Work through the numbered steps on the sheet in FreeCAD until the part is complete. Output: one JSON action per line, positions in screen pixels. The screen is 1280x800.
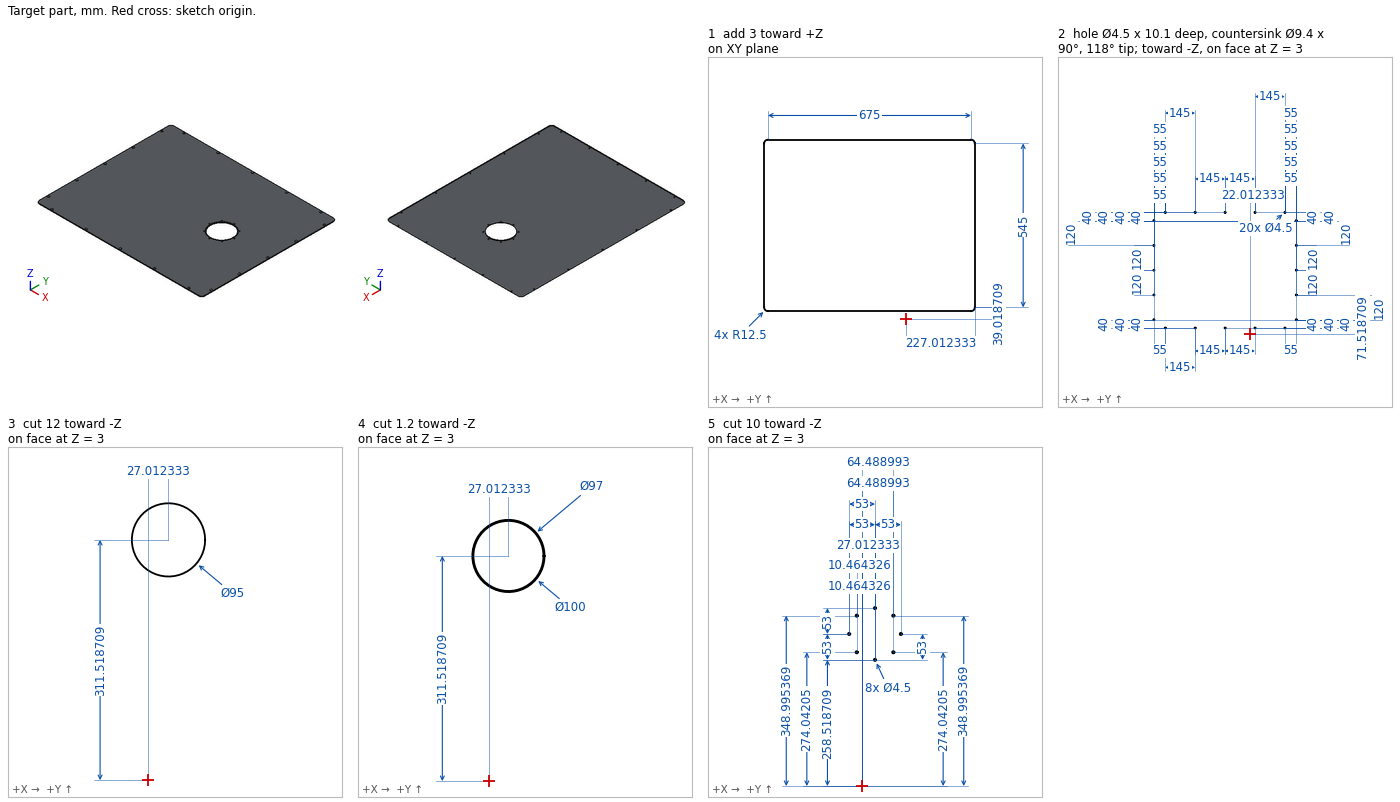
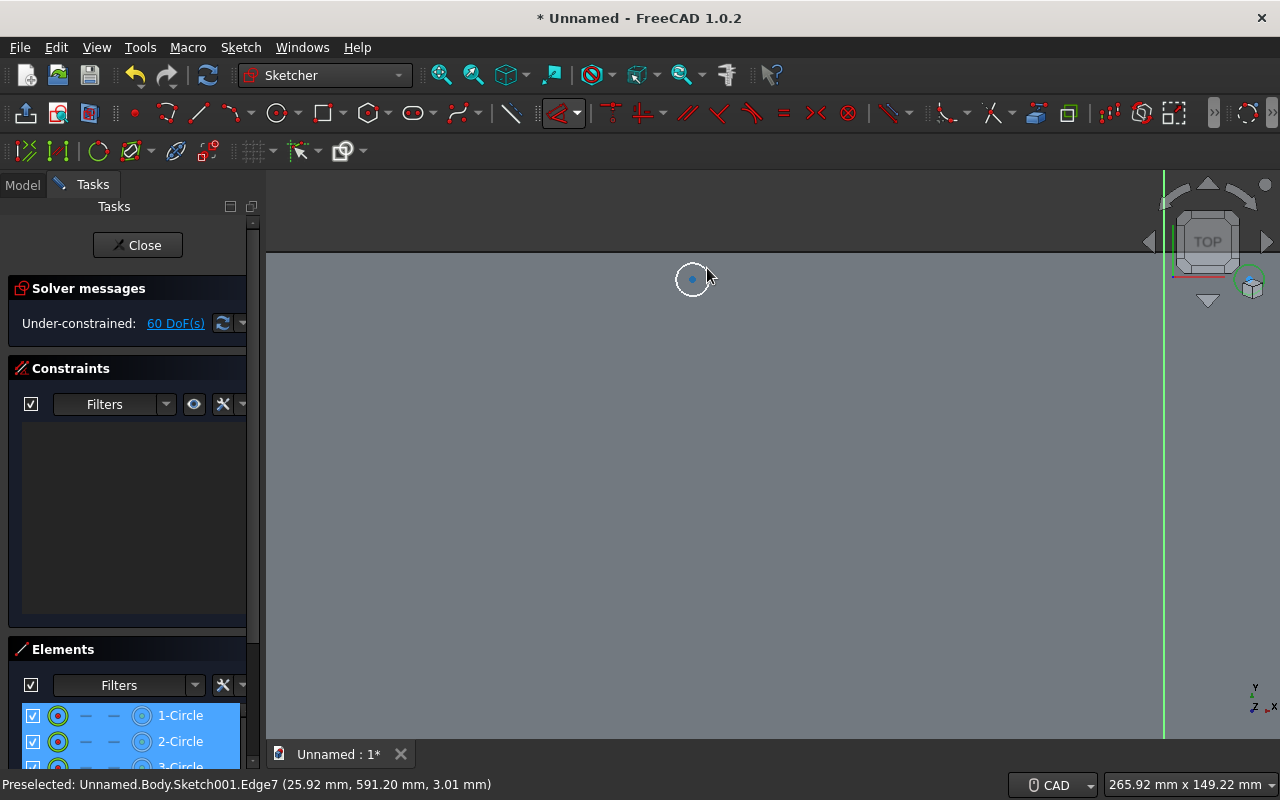
{"action": "left_click", "coordinate": [704, 268]}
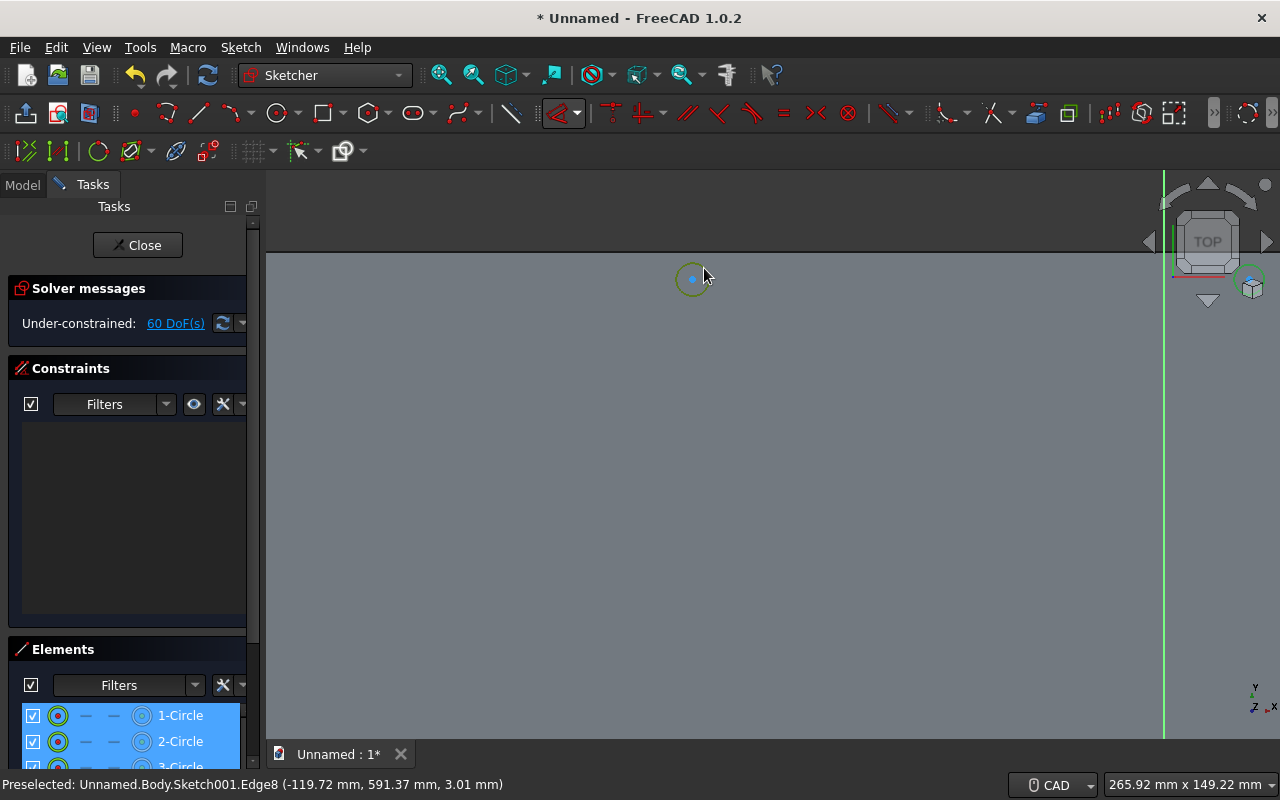
{"action": "scroll", "coordinate": [706, 268], "scroll_direction": "down", "scroll_amount": 9}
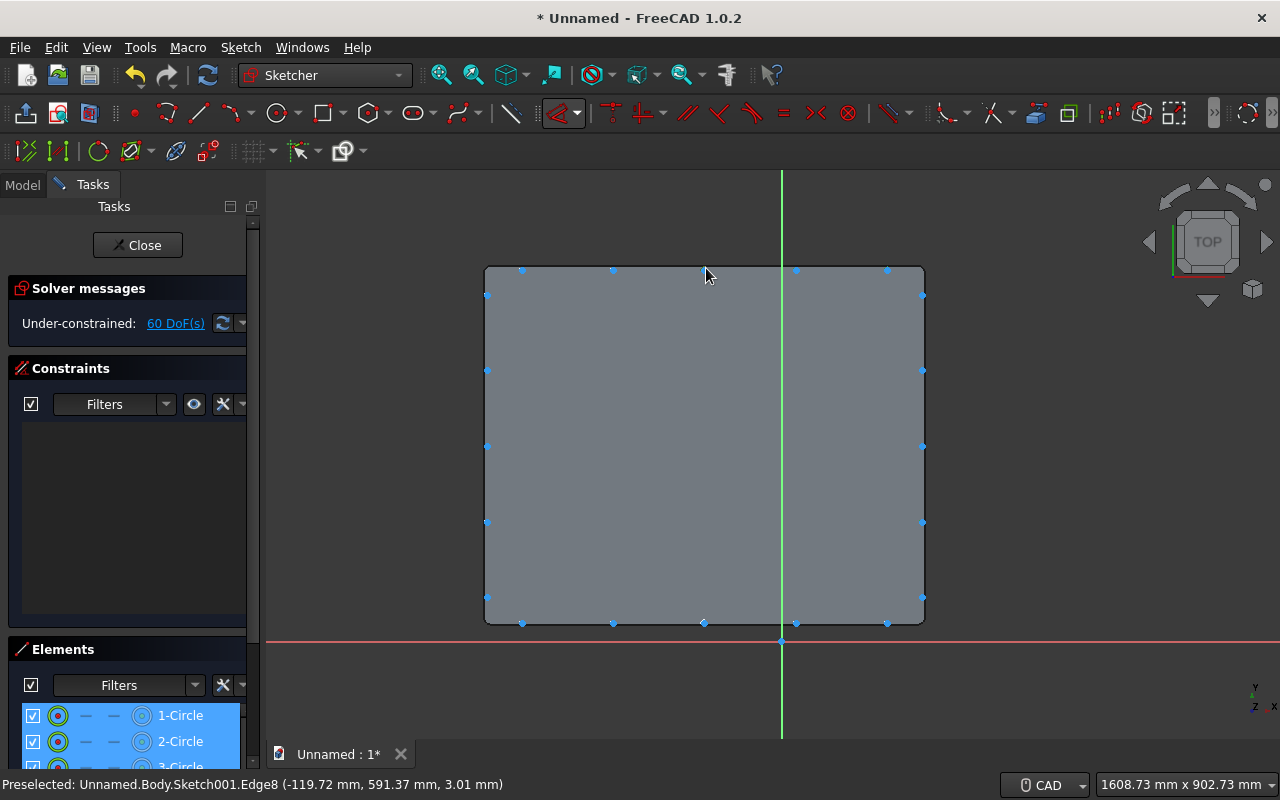
{"action": "scroll", "coordinate": [615, 268], "scroll_direction": "up", "scroll_amount": 9}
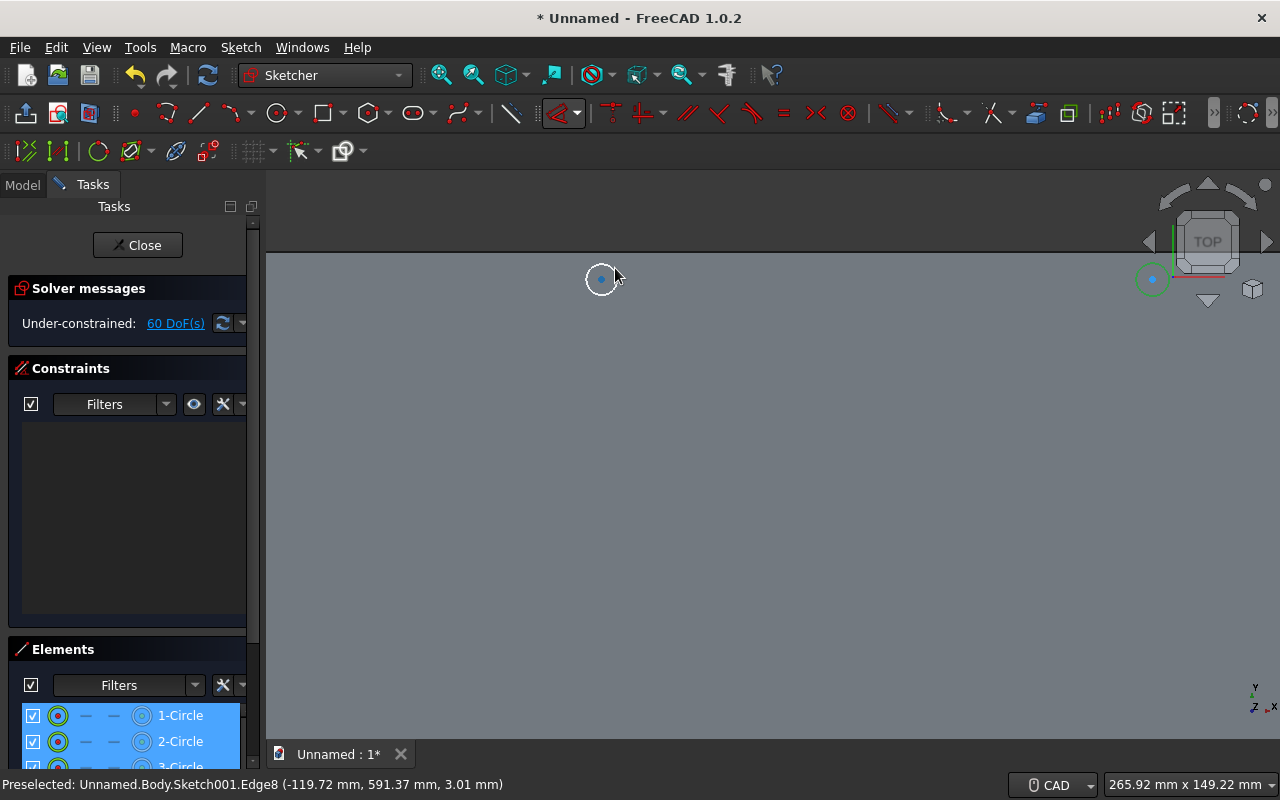
{"action": "left_click", "coordinate": [613, 269]}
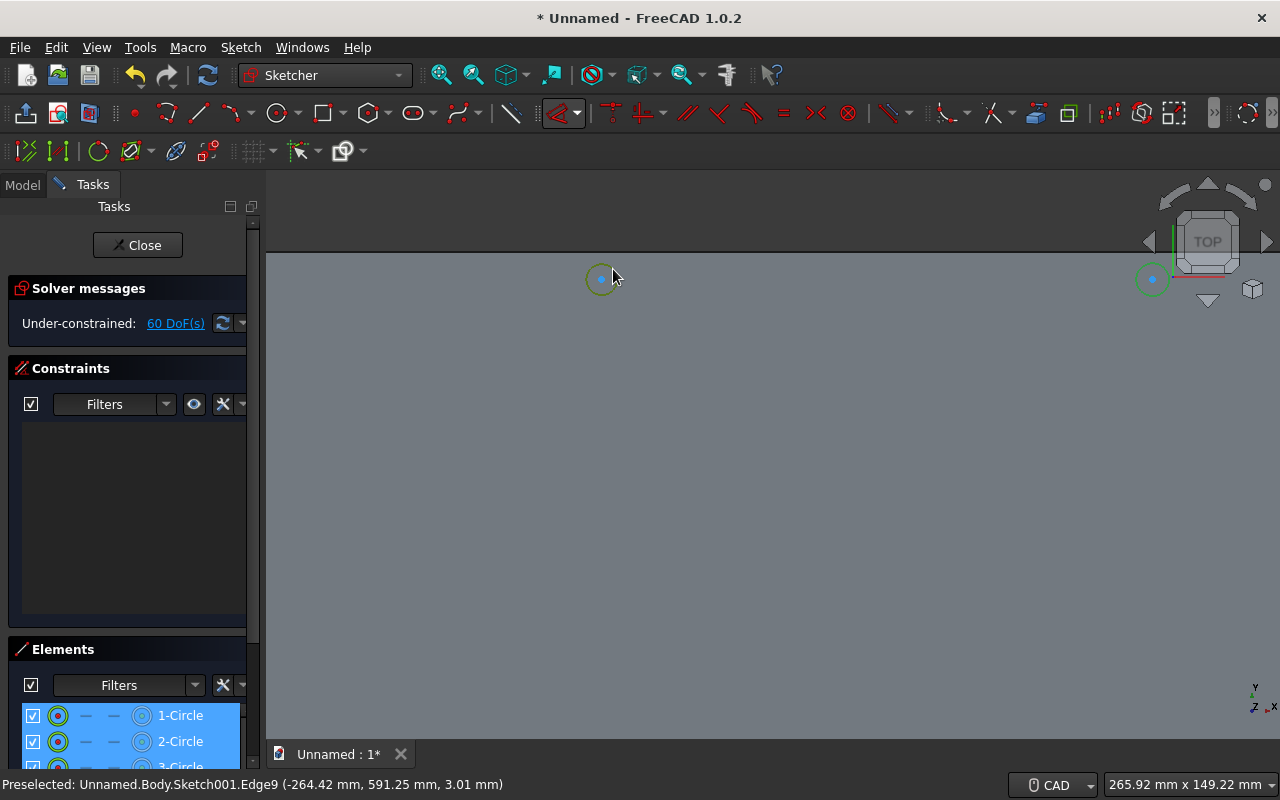
{"action": "scroll", "coordinate": [615, 268], "scroll_direction": "down", "scroll_amount": 9}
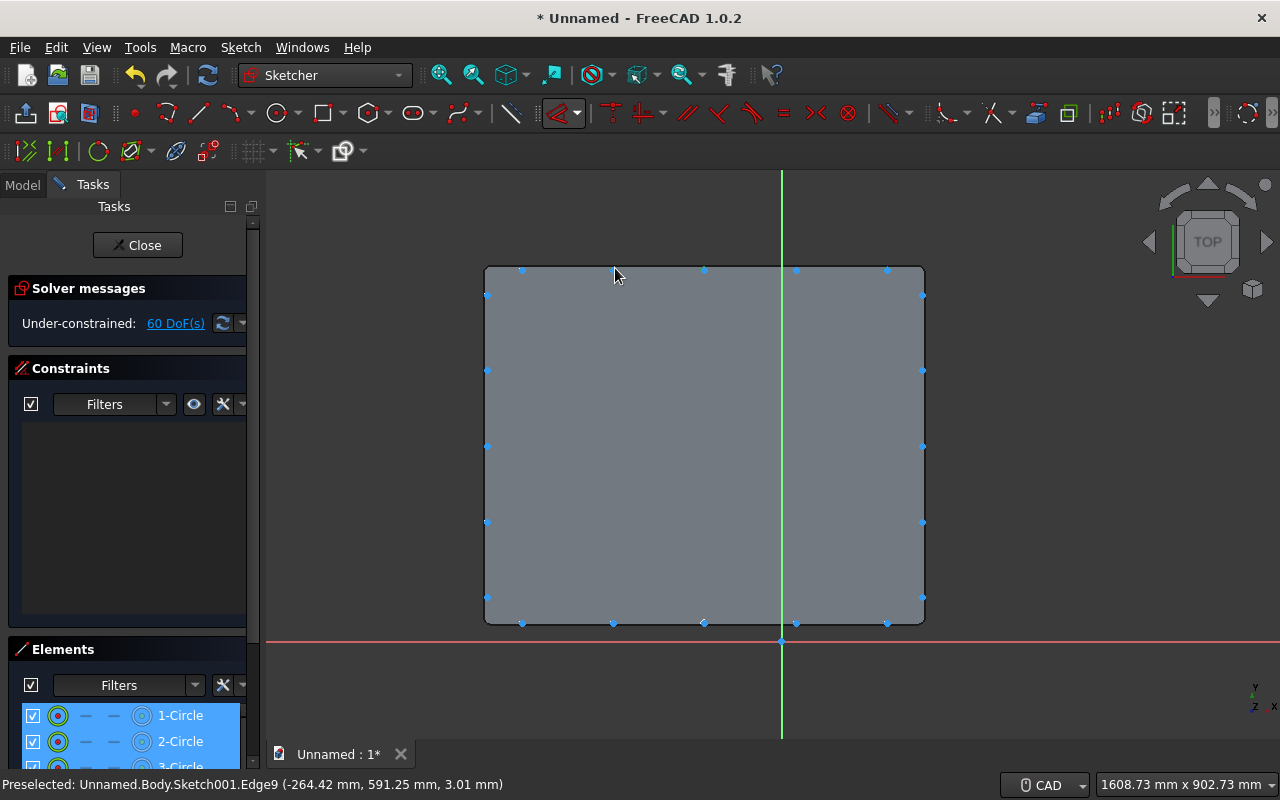
{"action": "scroll", "coordinate": [524, 268], "scroll_direction": "up", "scroll_amount": 9}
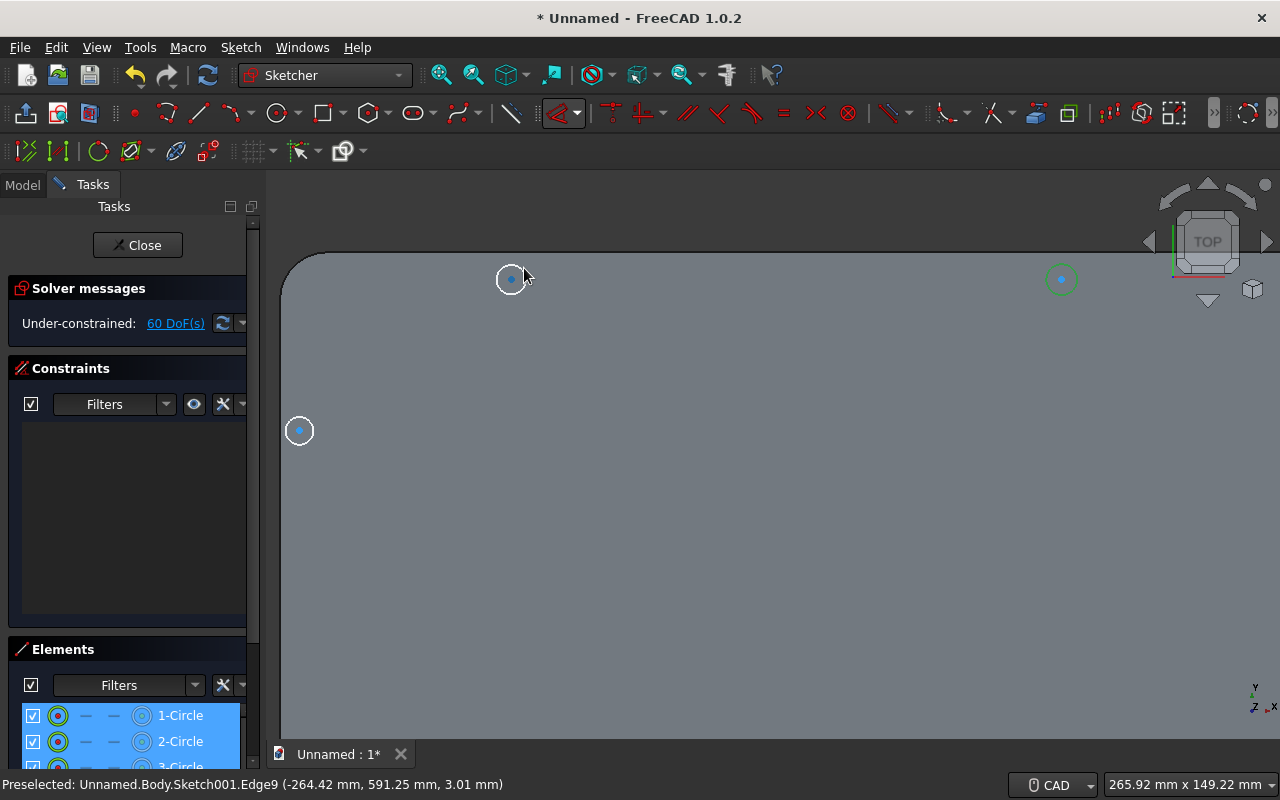
{"action": "left_click", "coordinate": [522, 269]}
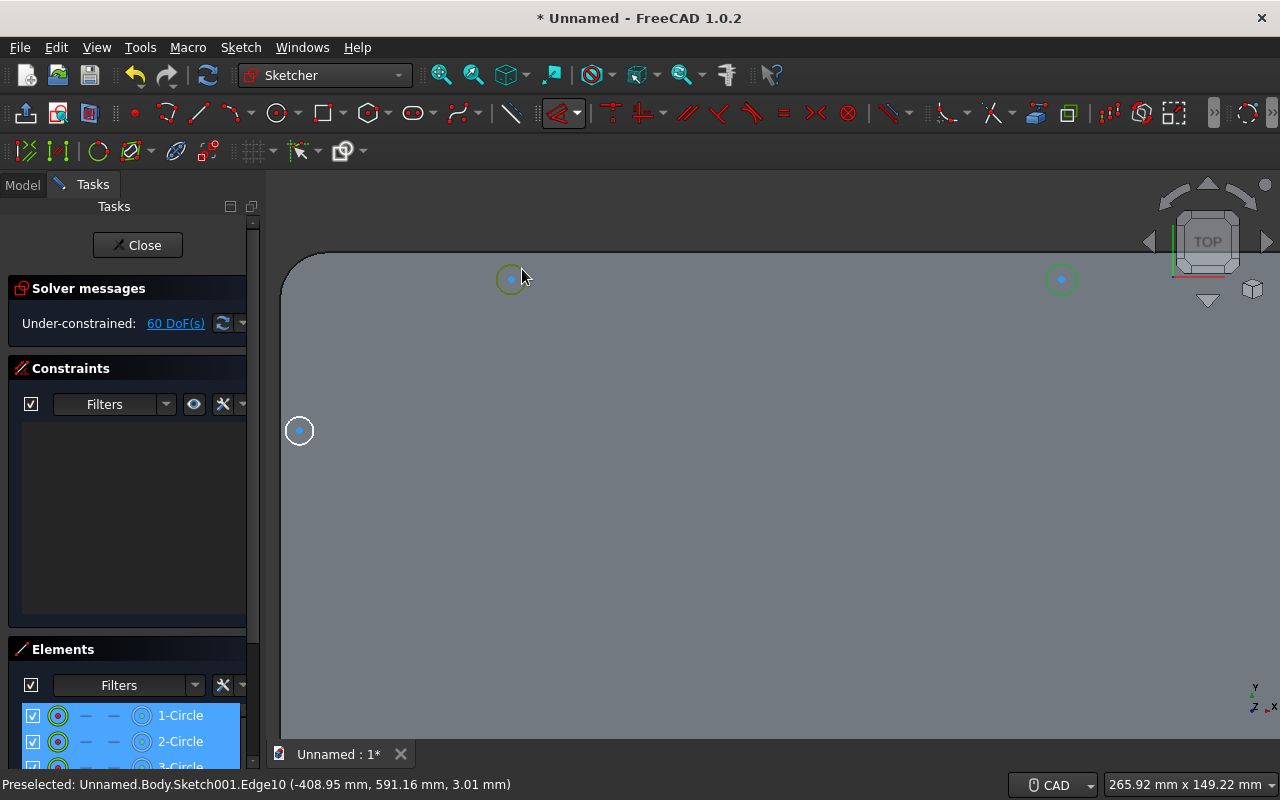
{"action": "left_click", "coordinate": [309, 421]}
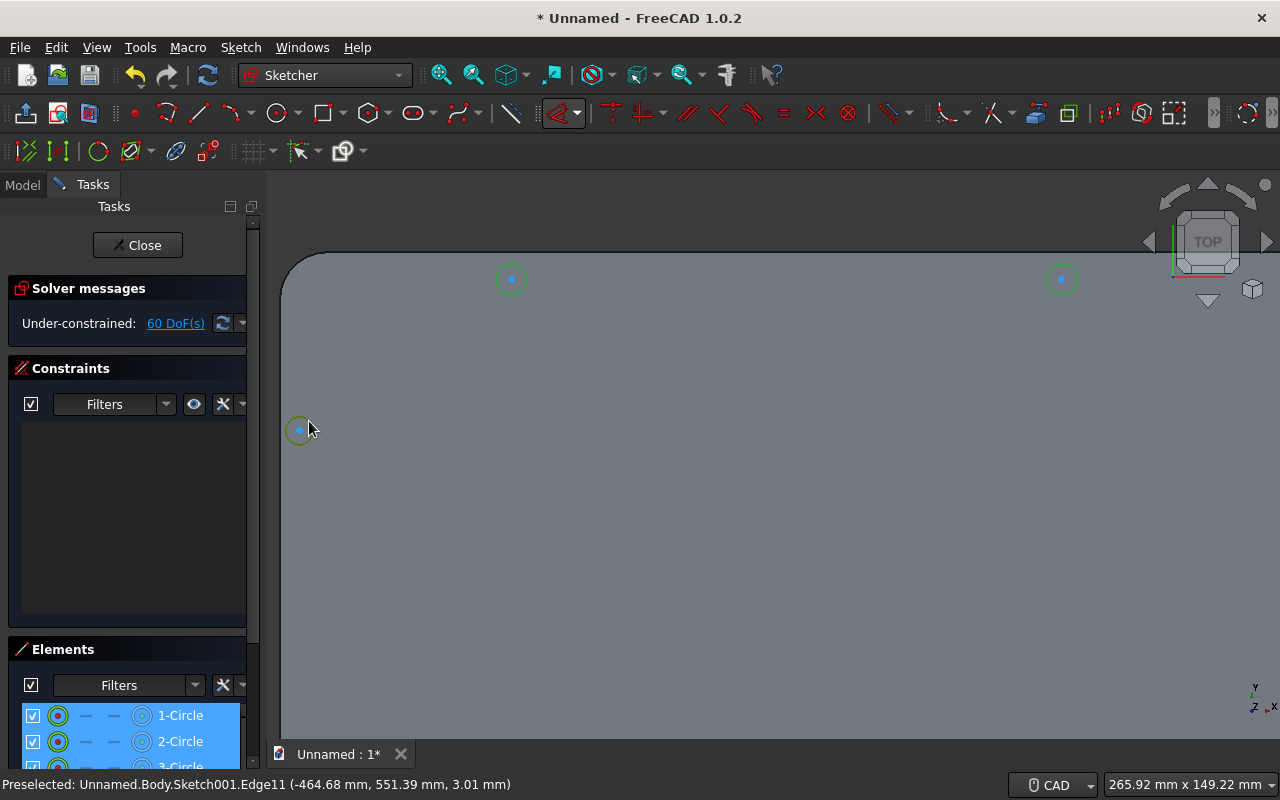
{"action": "scroll", "coordinate": [524, 268], "scroll_direction": "down", "scroll_amount": 9}